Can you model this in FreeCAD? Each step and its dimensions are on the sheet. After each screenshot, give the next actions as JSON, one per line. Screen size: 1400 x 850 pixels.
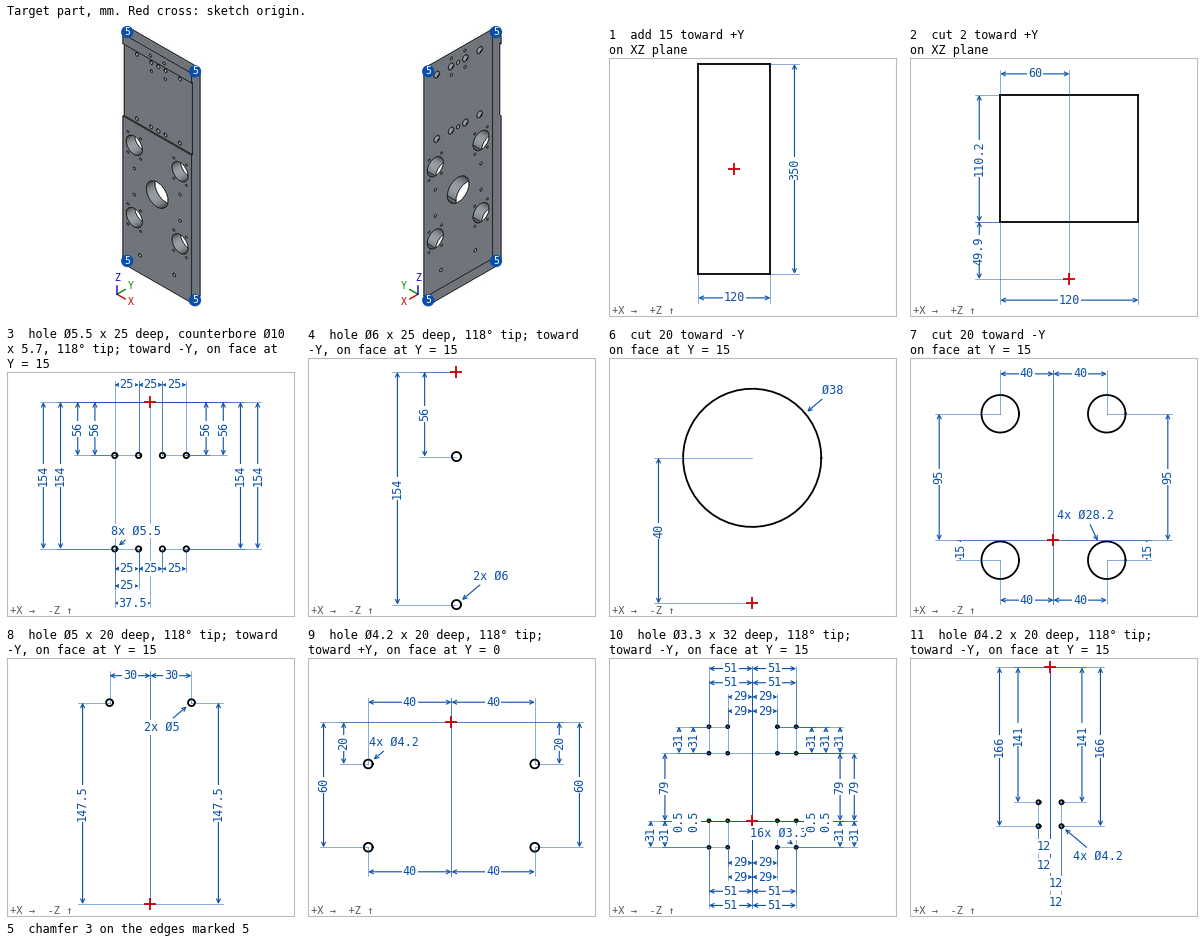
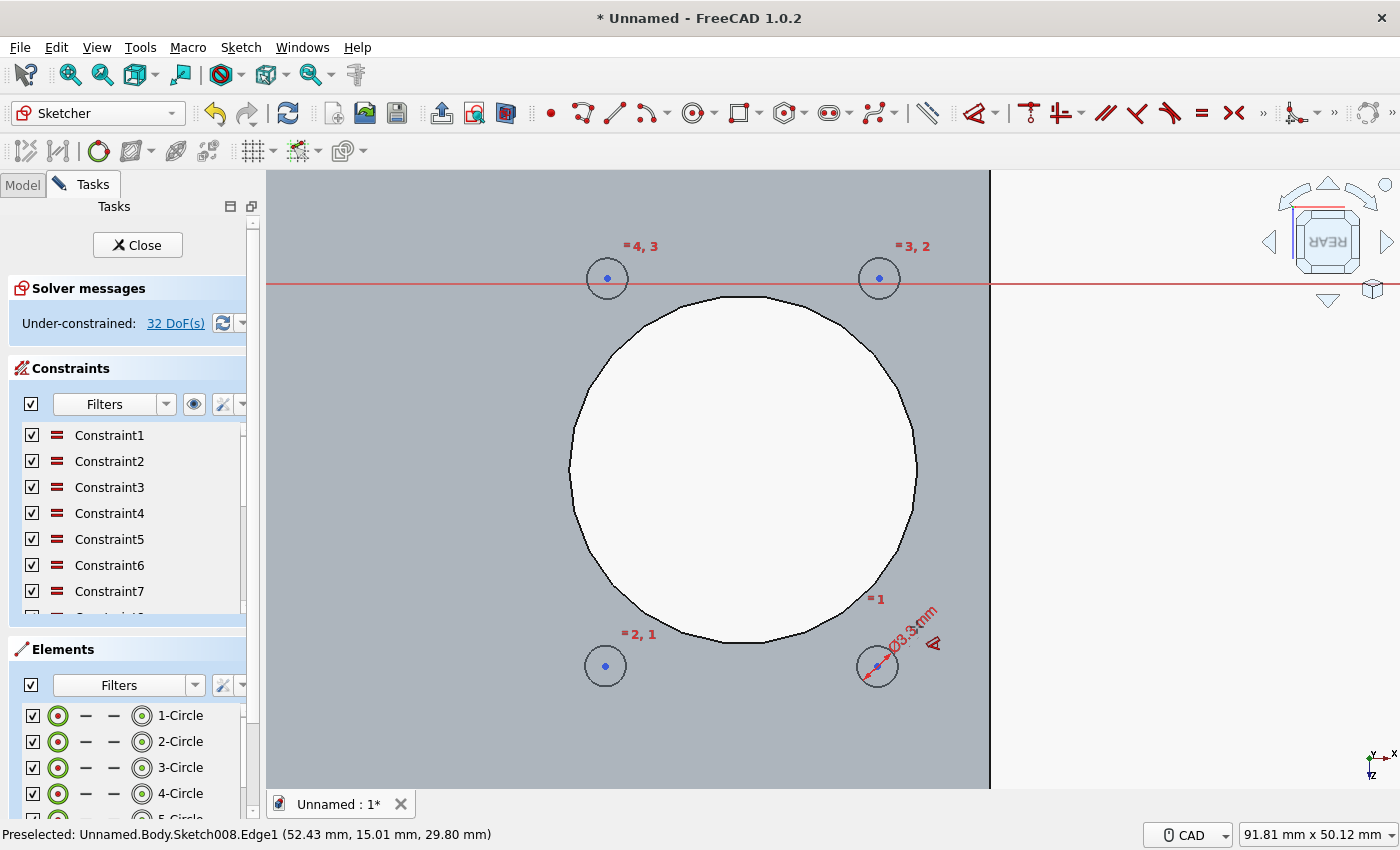
{"action": "scroll", "coordinate": [895, 654], "scroll_direction": "down", "scroll_amount": 8}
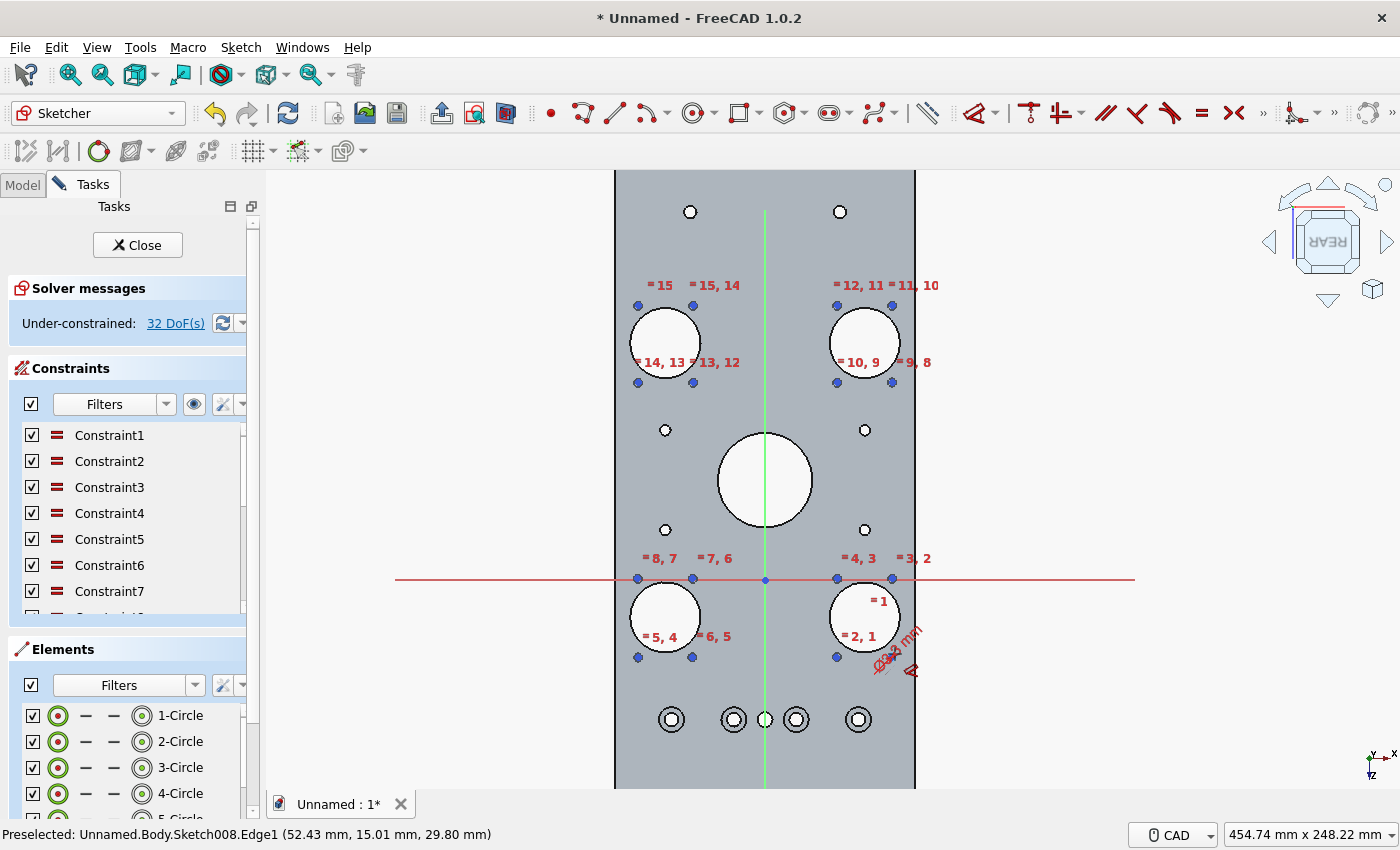
{"action": "left_click", "coordinate": [892, 657]}
{"action": "left_click", "coordinate": [828, 691]}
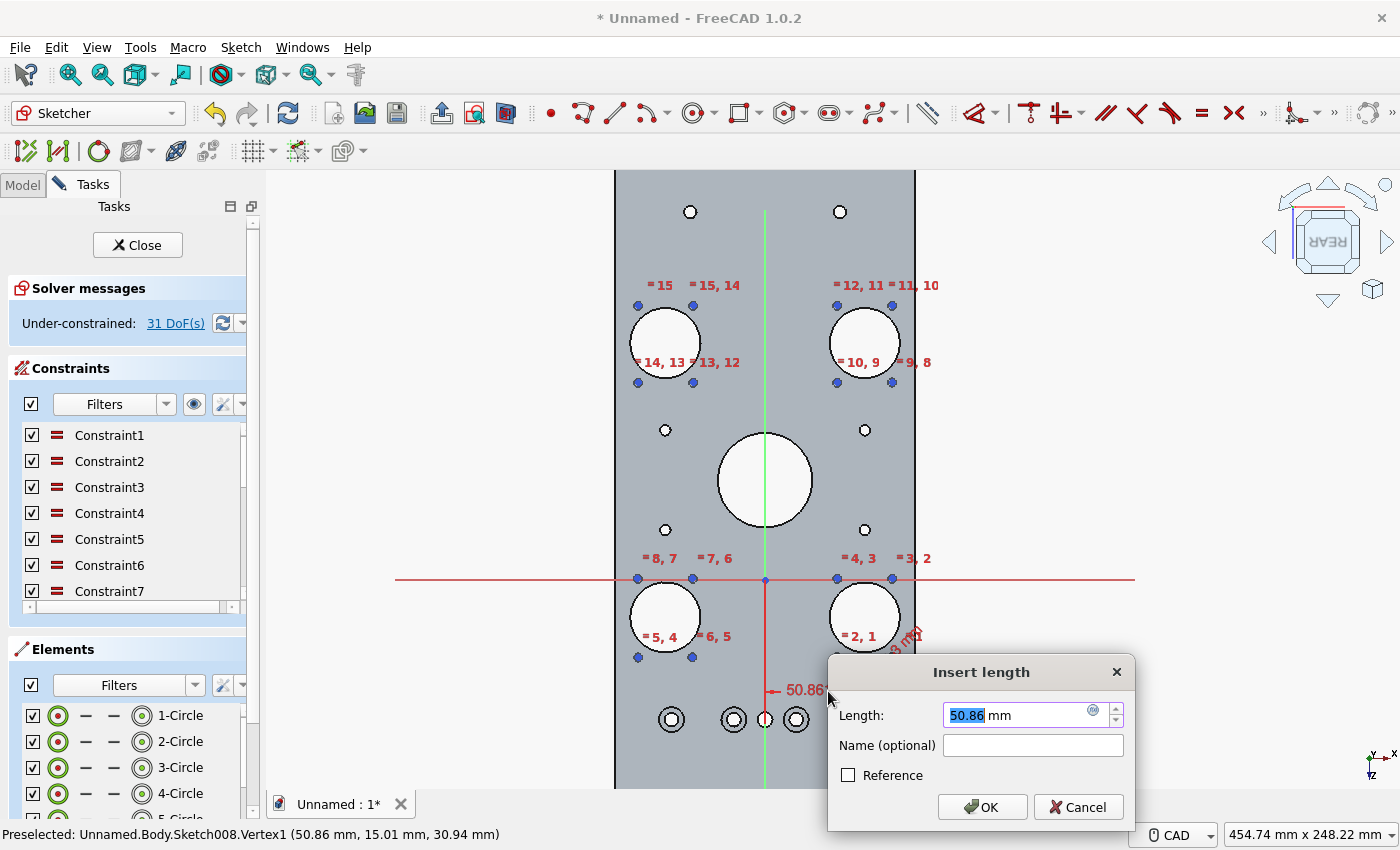
{"action": "type", "text": "51"}
{"action": "key", "text": "Return"}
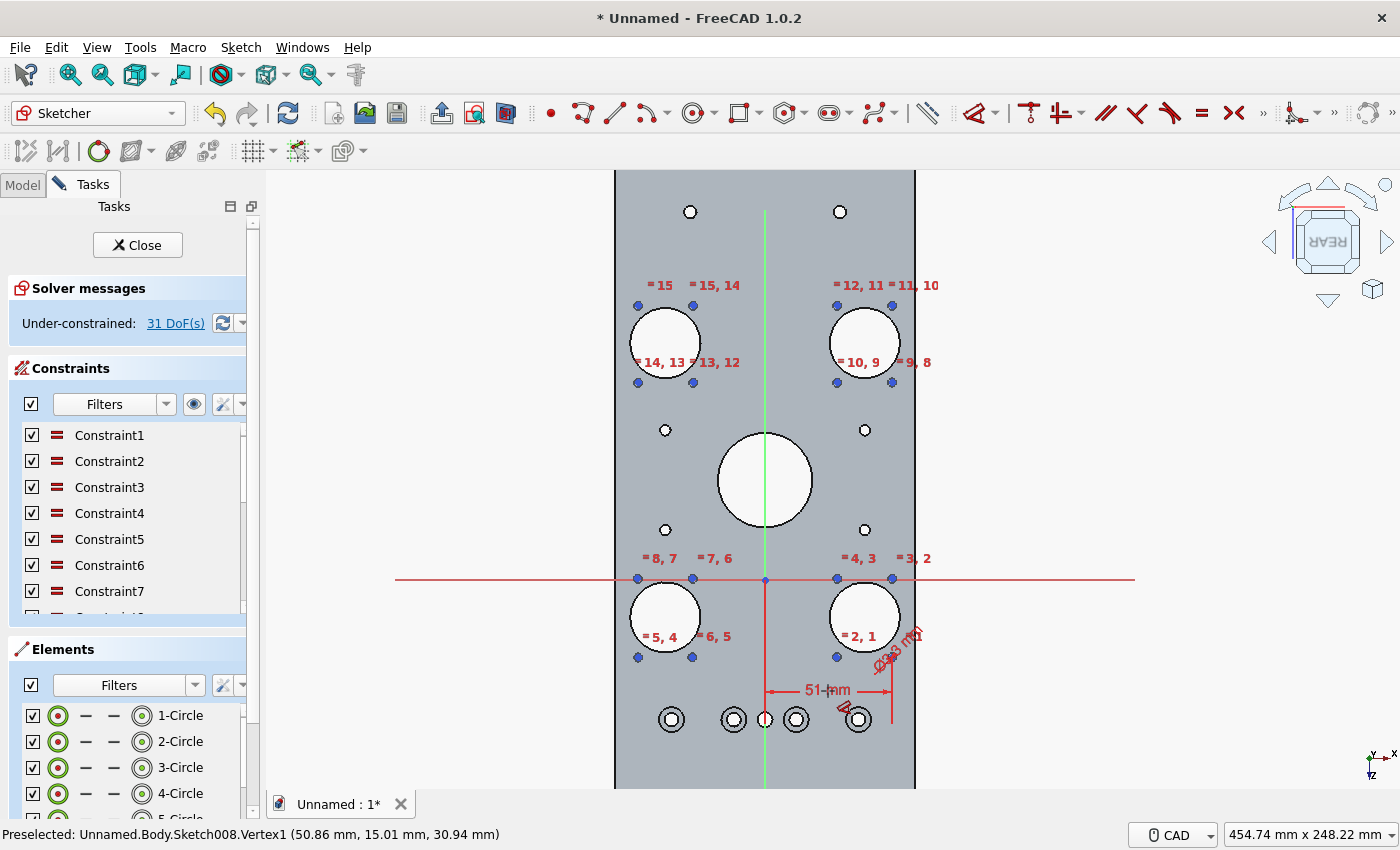
{"action": "left_click", "coordinate": [837, 657]}
{"action": "left_click", "coordinate": [801, 546]}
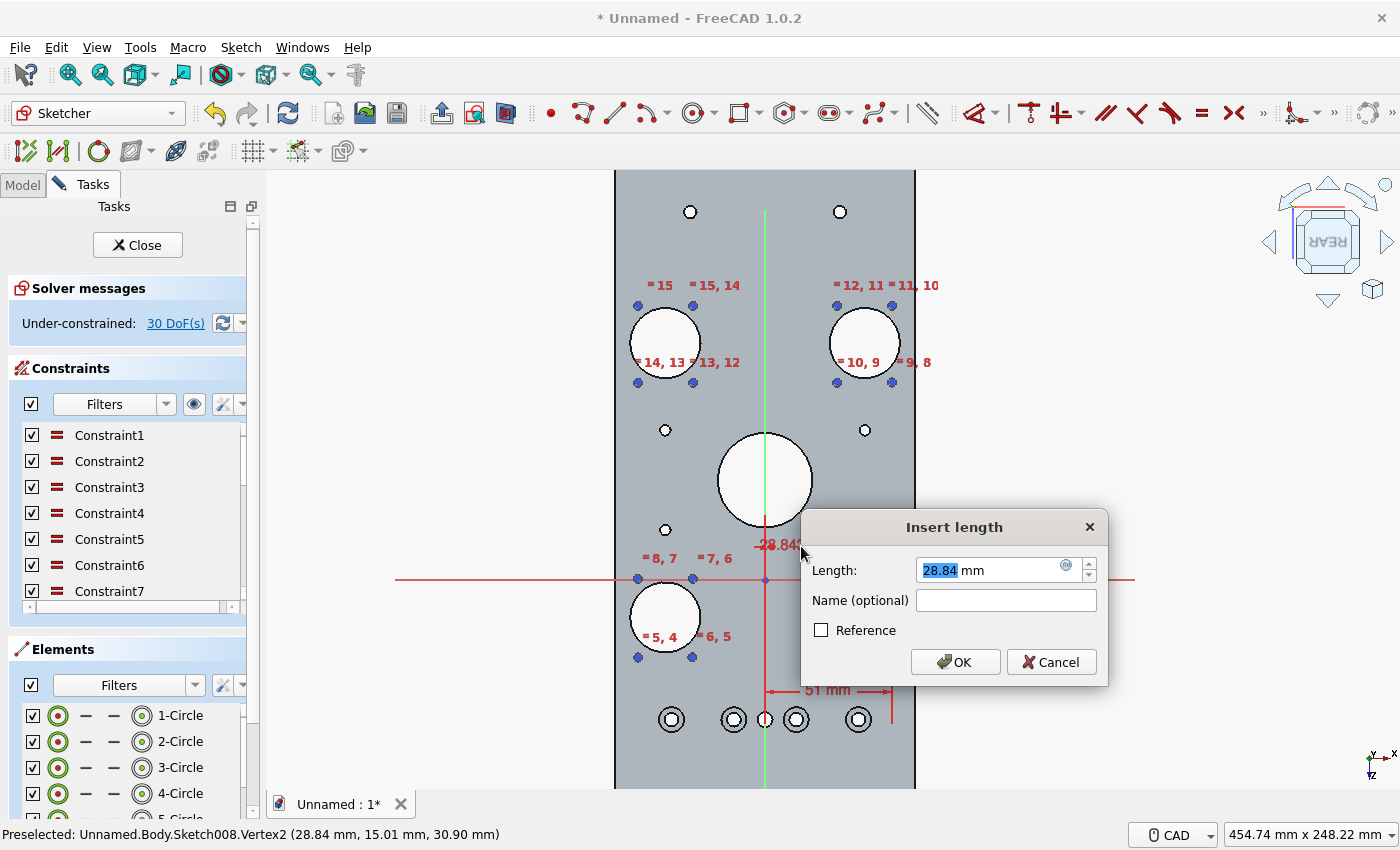
{"action": "type", "text": "29"}
{"action": "key", "text": "Return"}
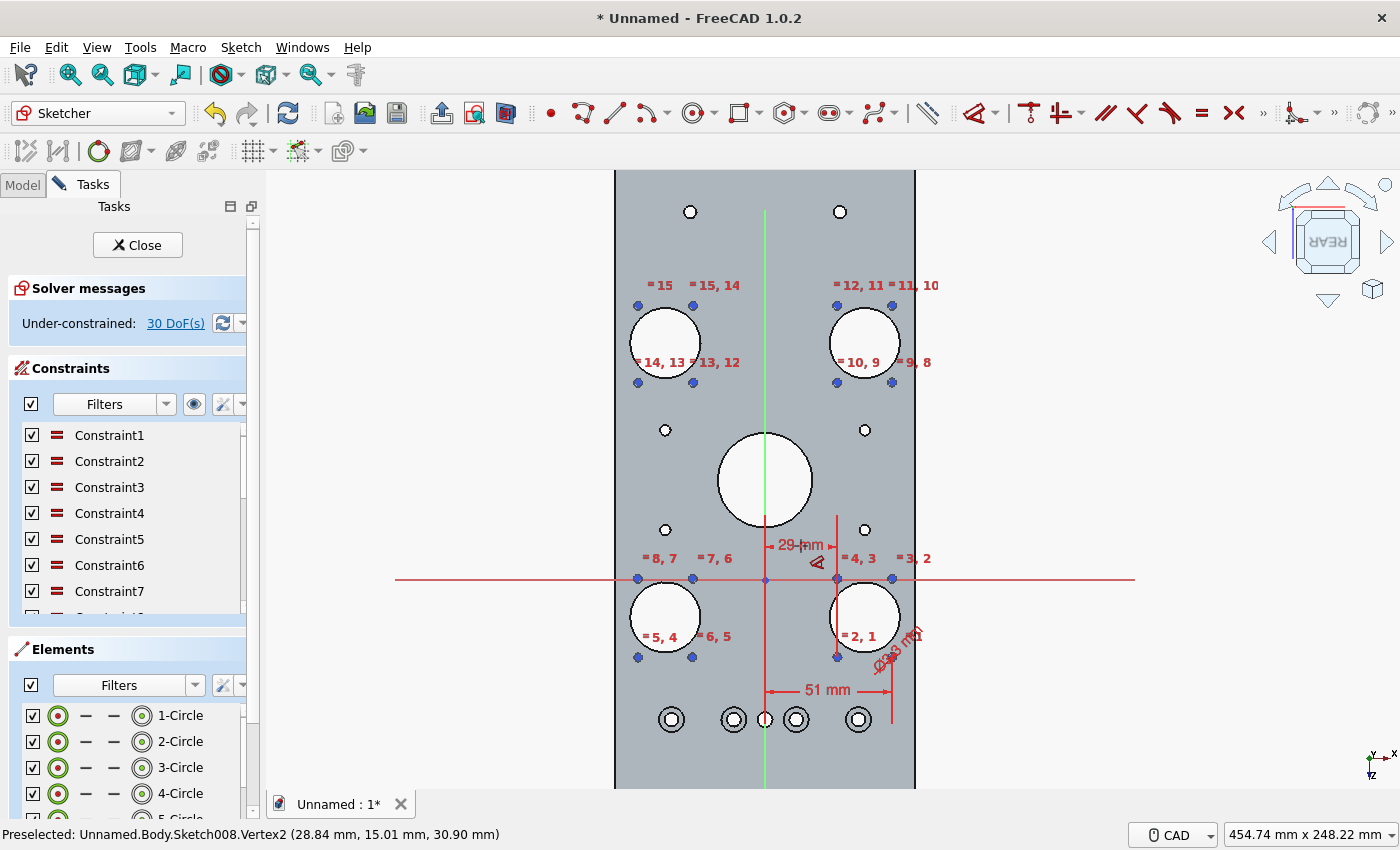
{"action": "left_click", "coordinate": [892, 579]}
{"action": "left_click", "coordinate": [829, 614]}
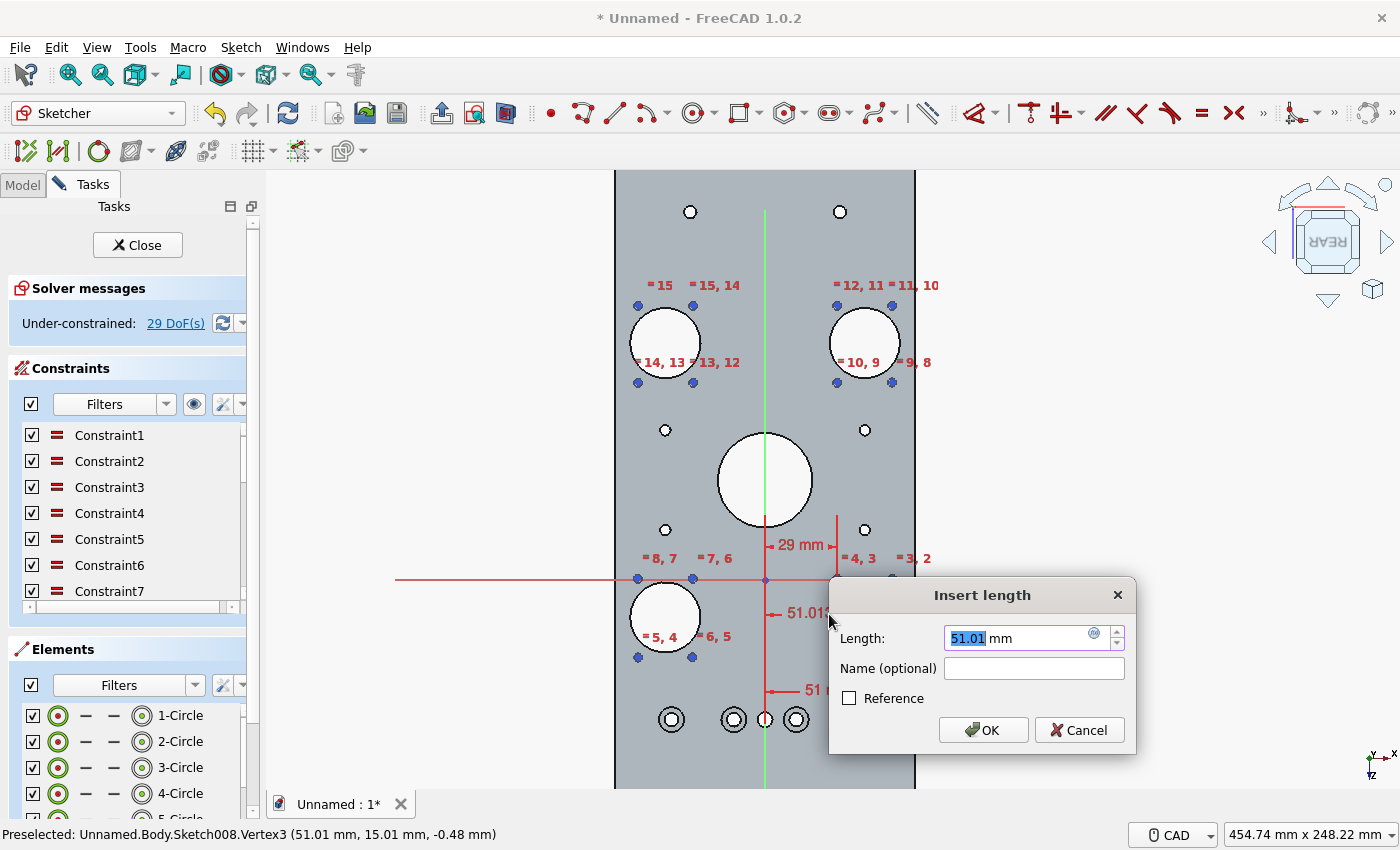
{"action": "type", "text": "51"}
{"action": "key", "text": "Return"}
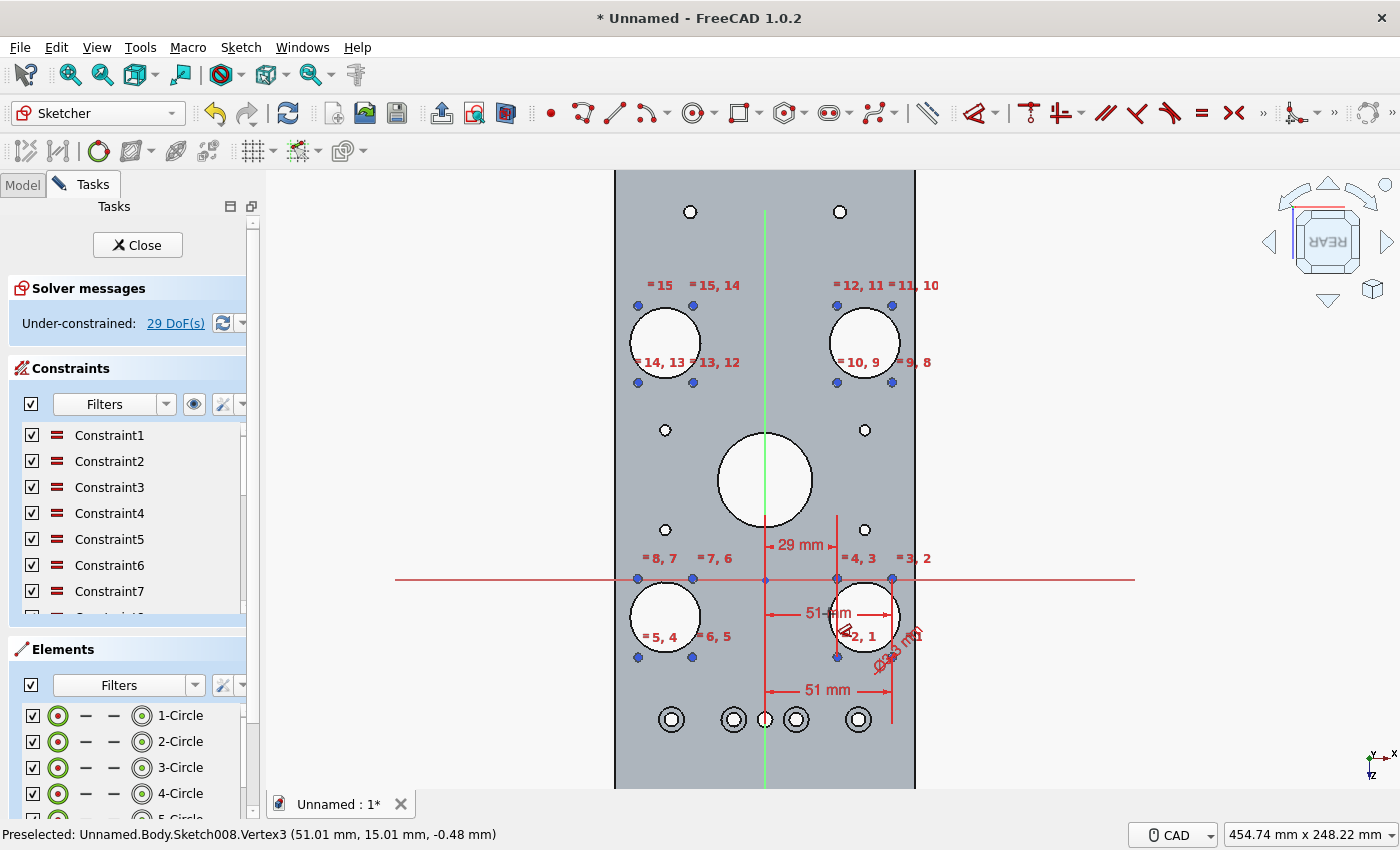
{"action": "left_click", "coordinate": [837, 579]}
{"action": "left_click", "coordinate": [801, 638]}